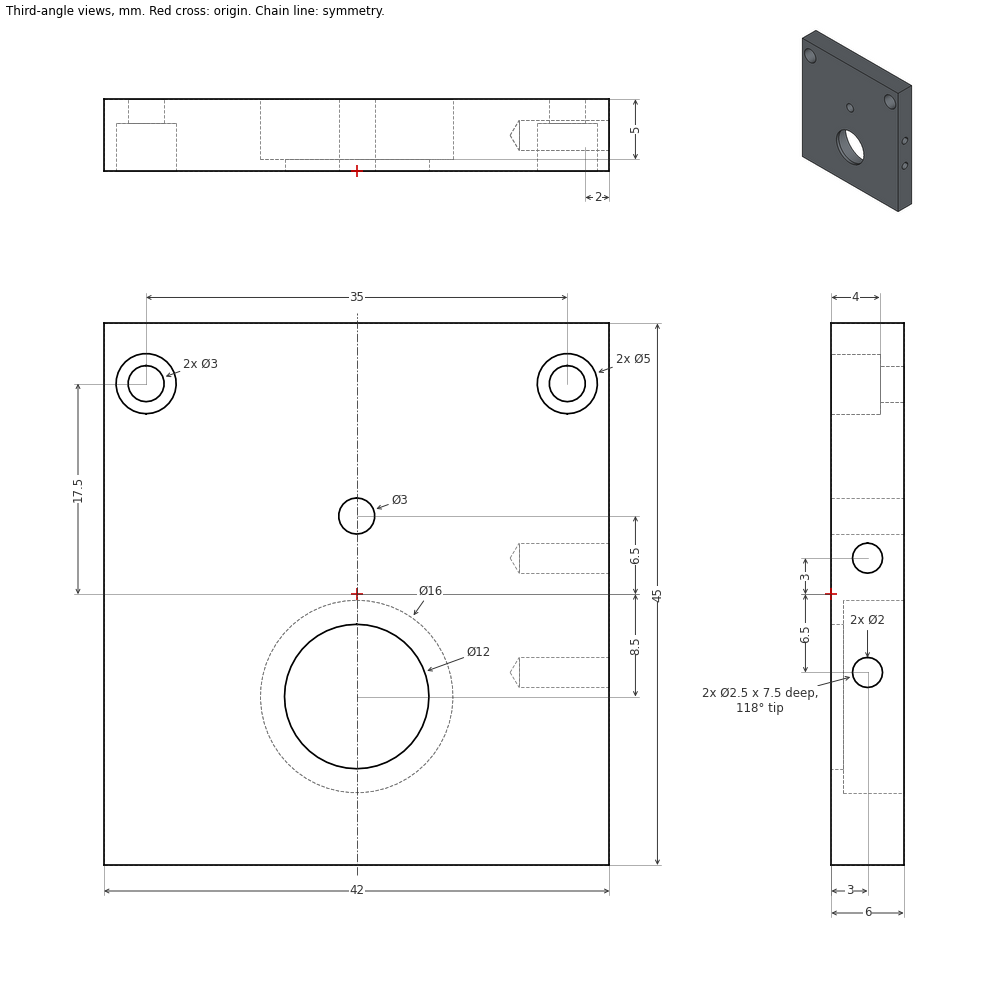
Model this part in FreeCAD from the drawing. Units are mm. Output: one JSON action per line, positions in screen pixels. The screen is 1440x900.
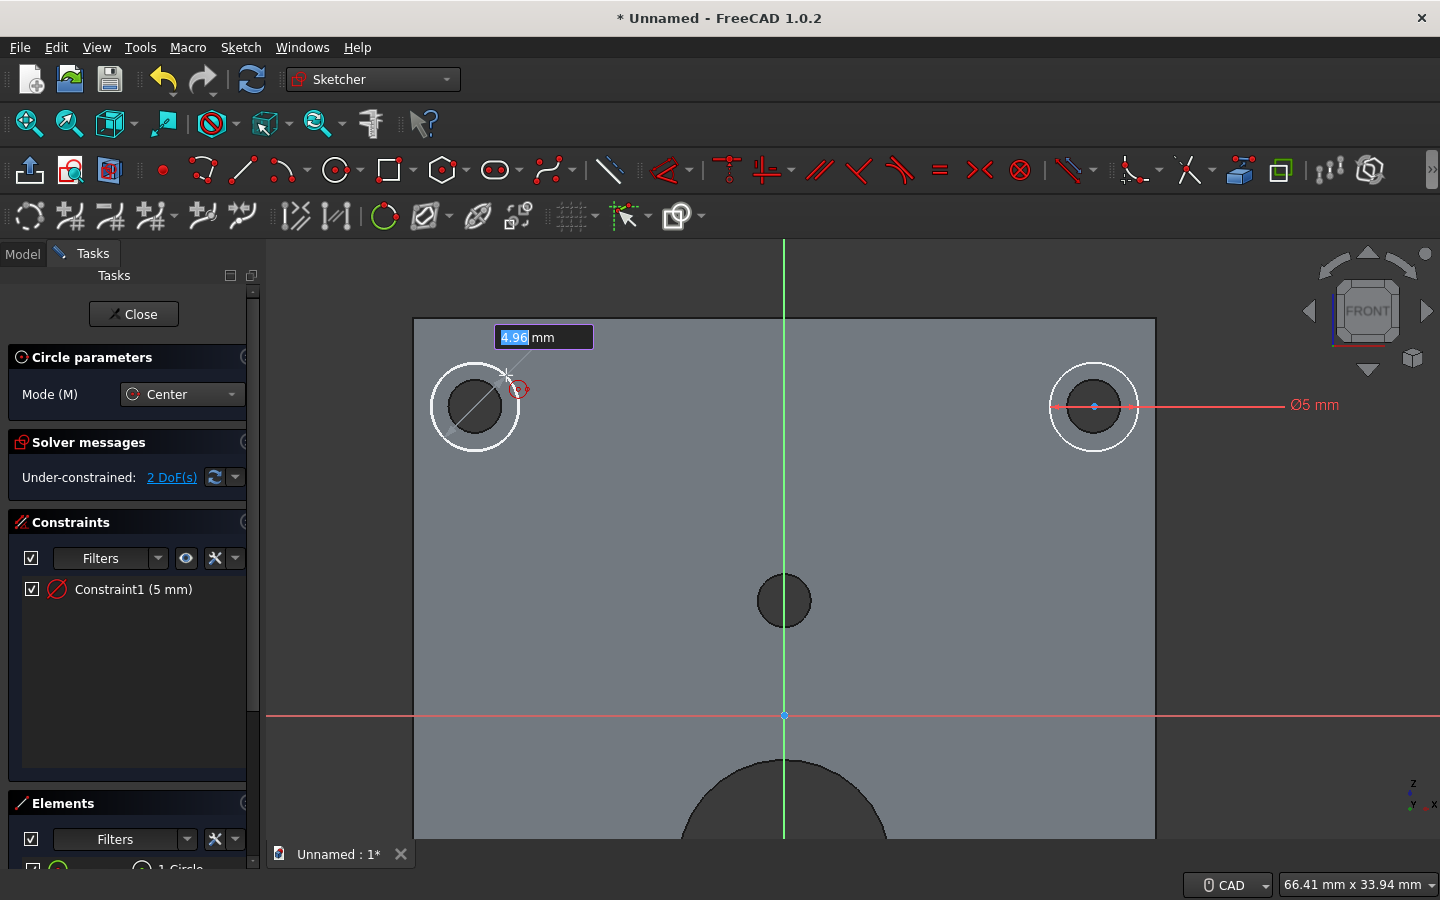
{"action": "type", "text": "5"}
{"action": "key", "text": "Return"}
{"action": "key", "text": "Escape"}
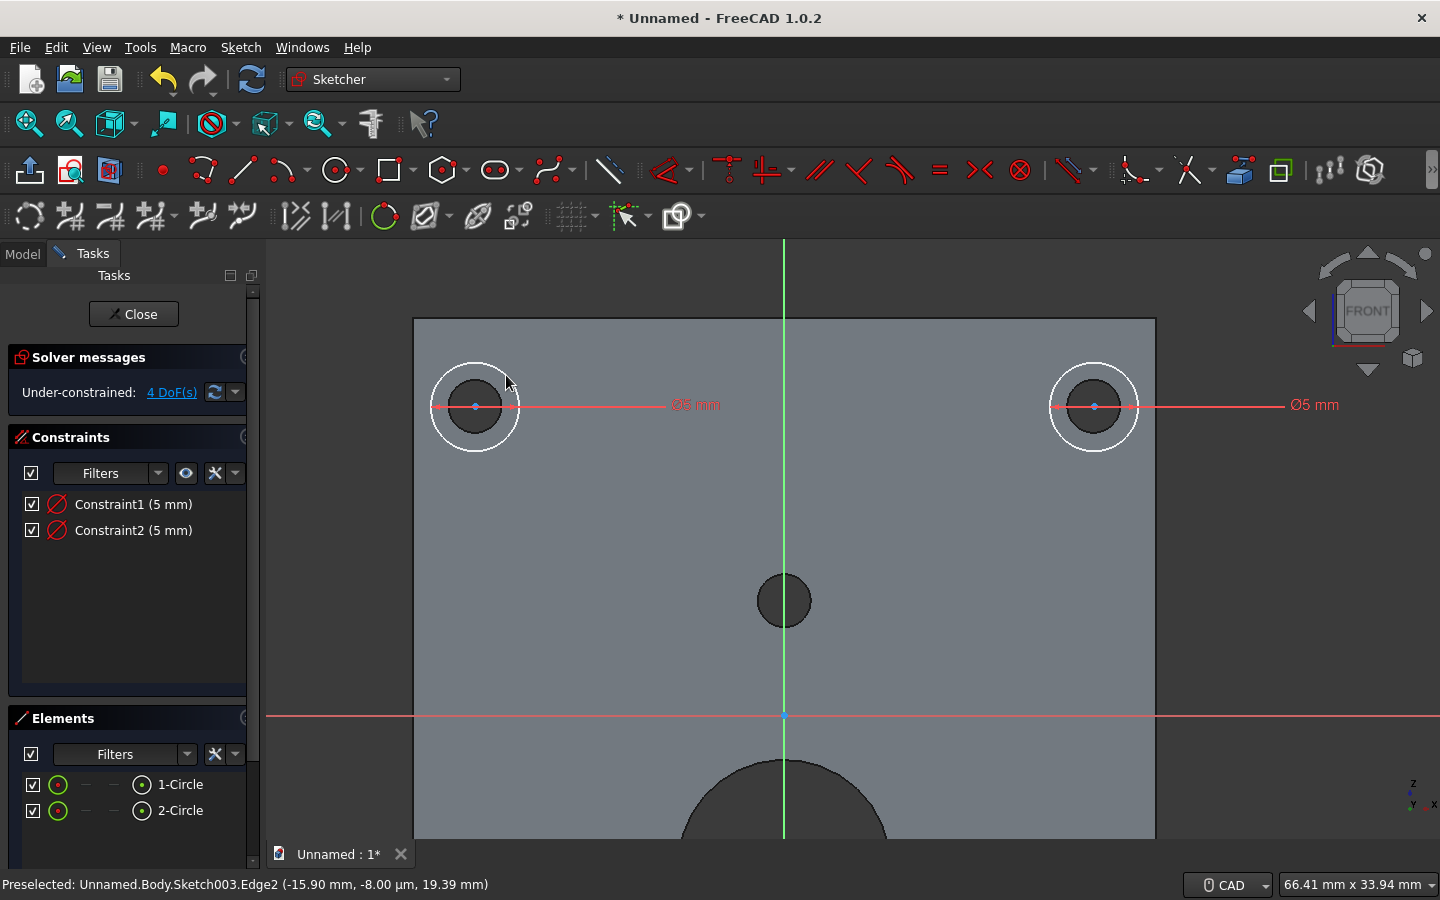
{"action": "left_click", "coordinate": [1094, 407]}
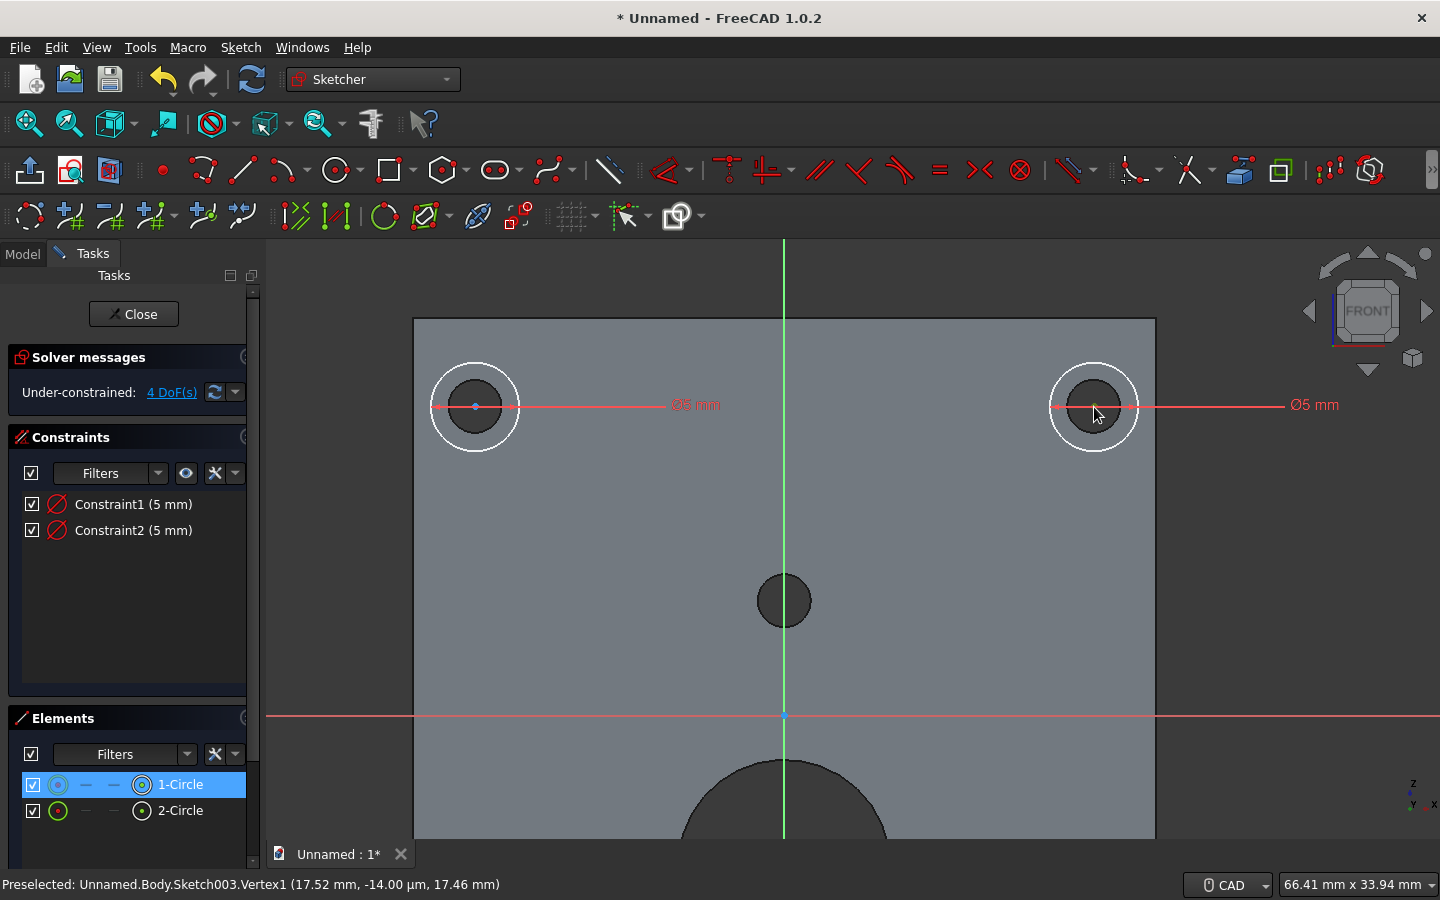
{"action": "left_click", "coordinate": [475, 407]}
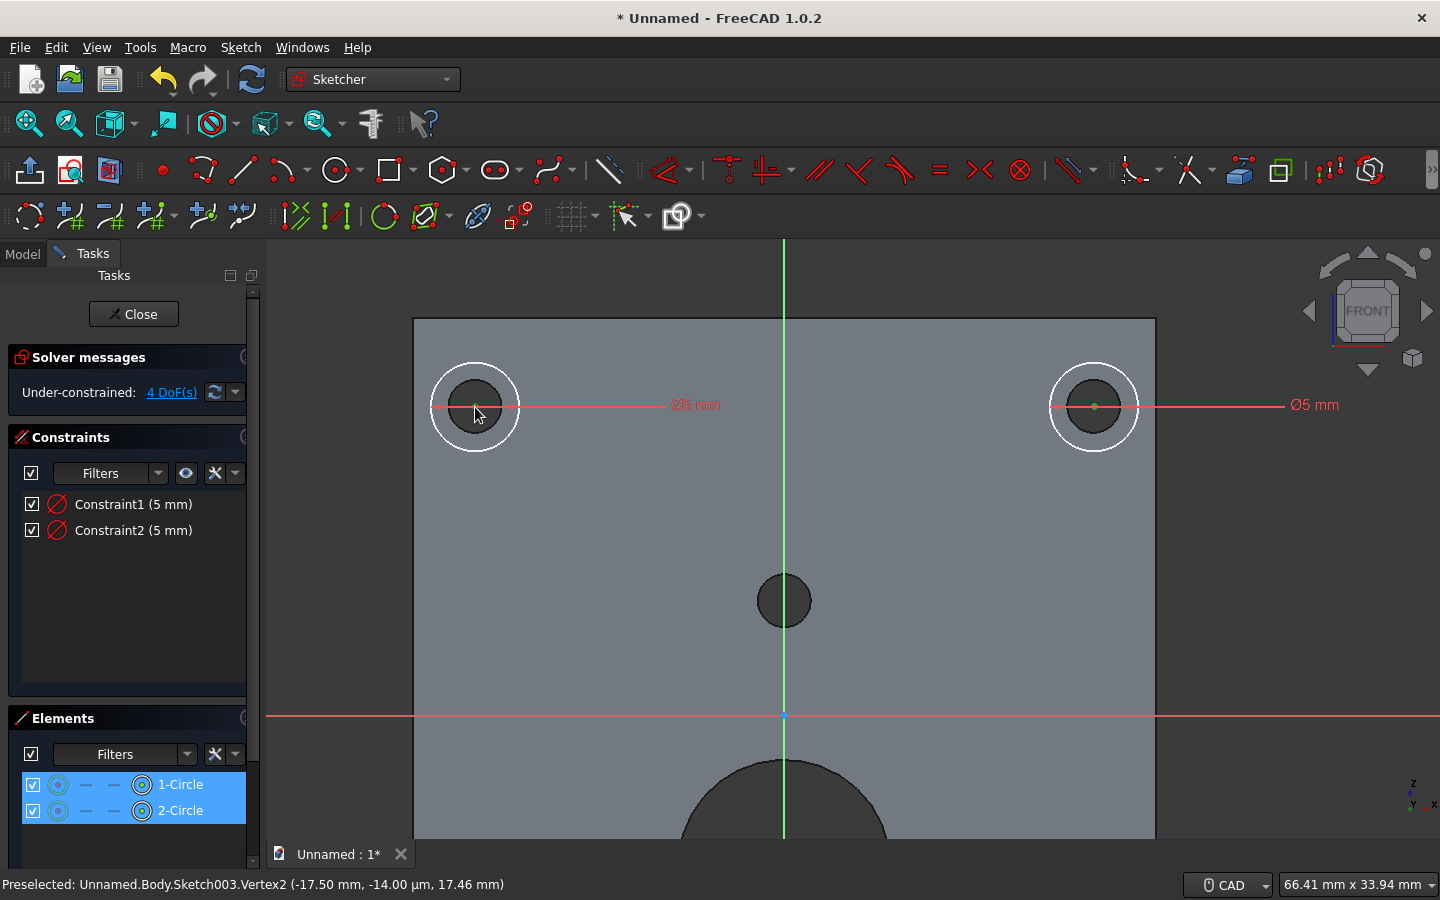
{"action": "left_click", "coordinate": [784, 772]}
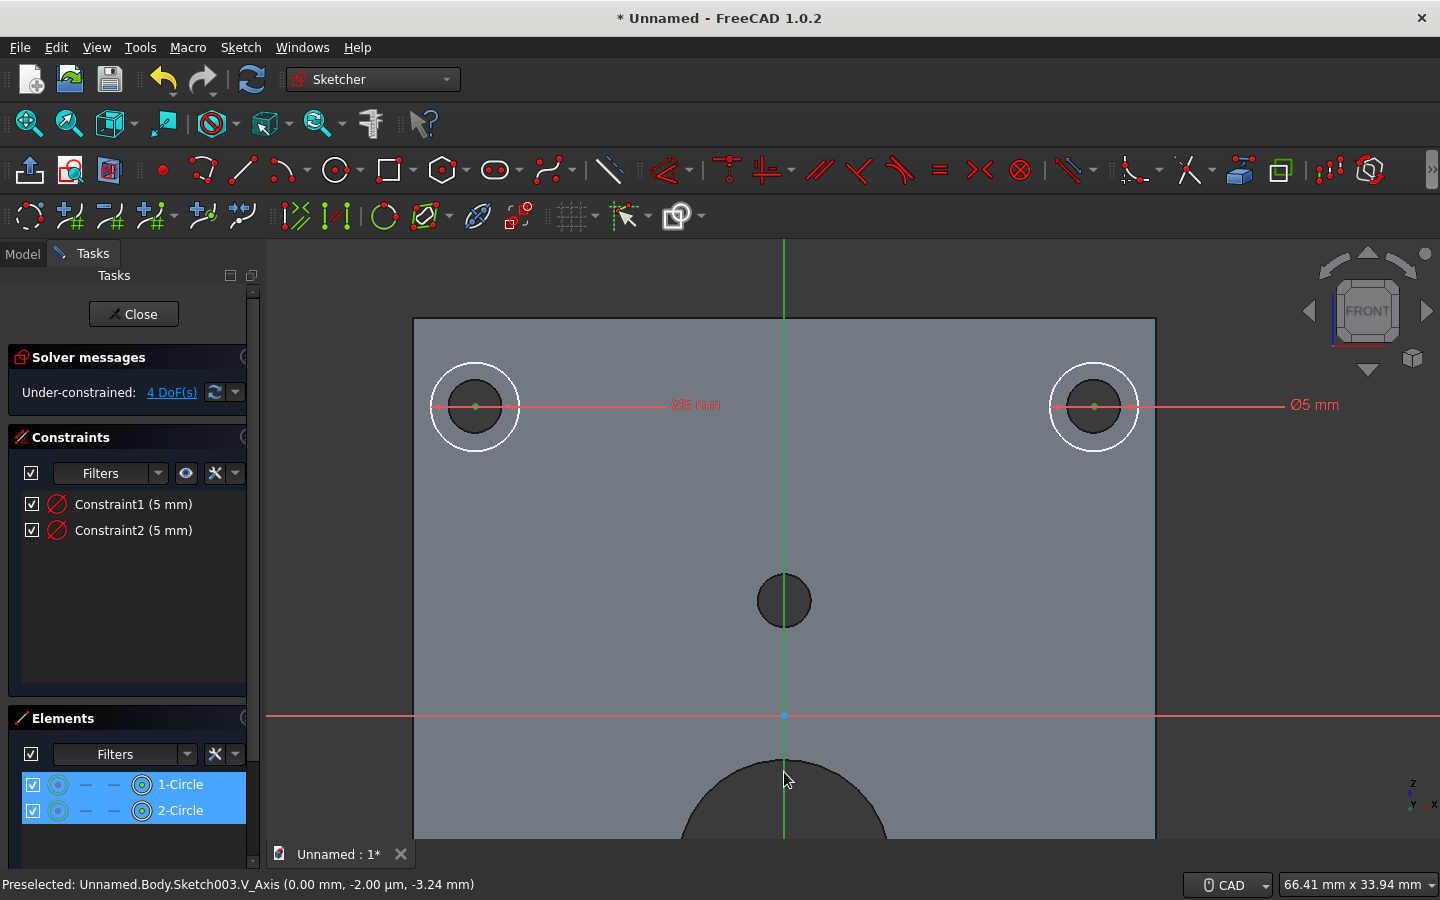
{"action": "key", "text": "s"}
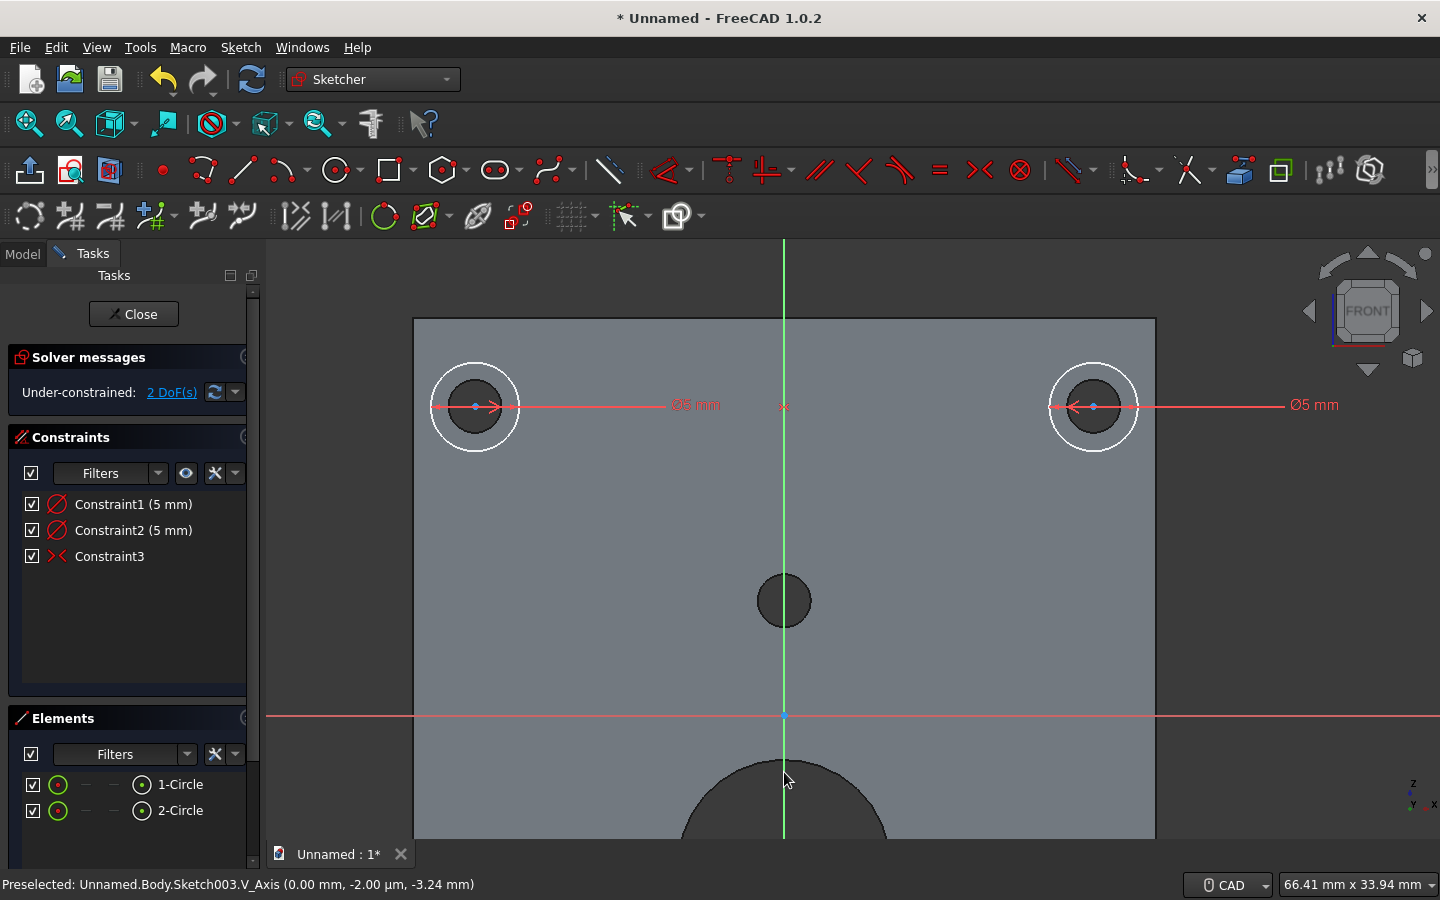
{"action": "key", "text": "d"}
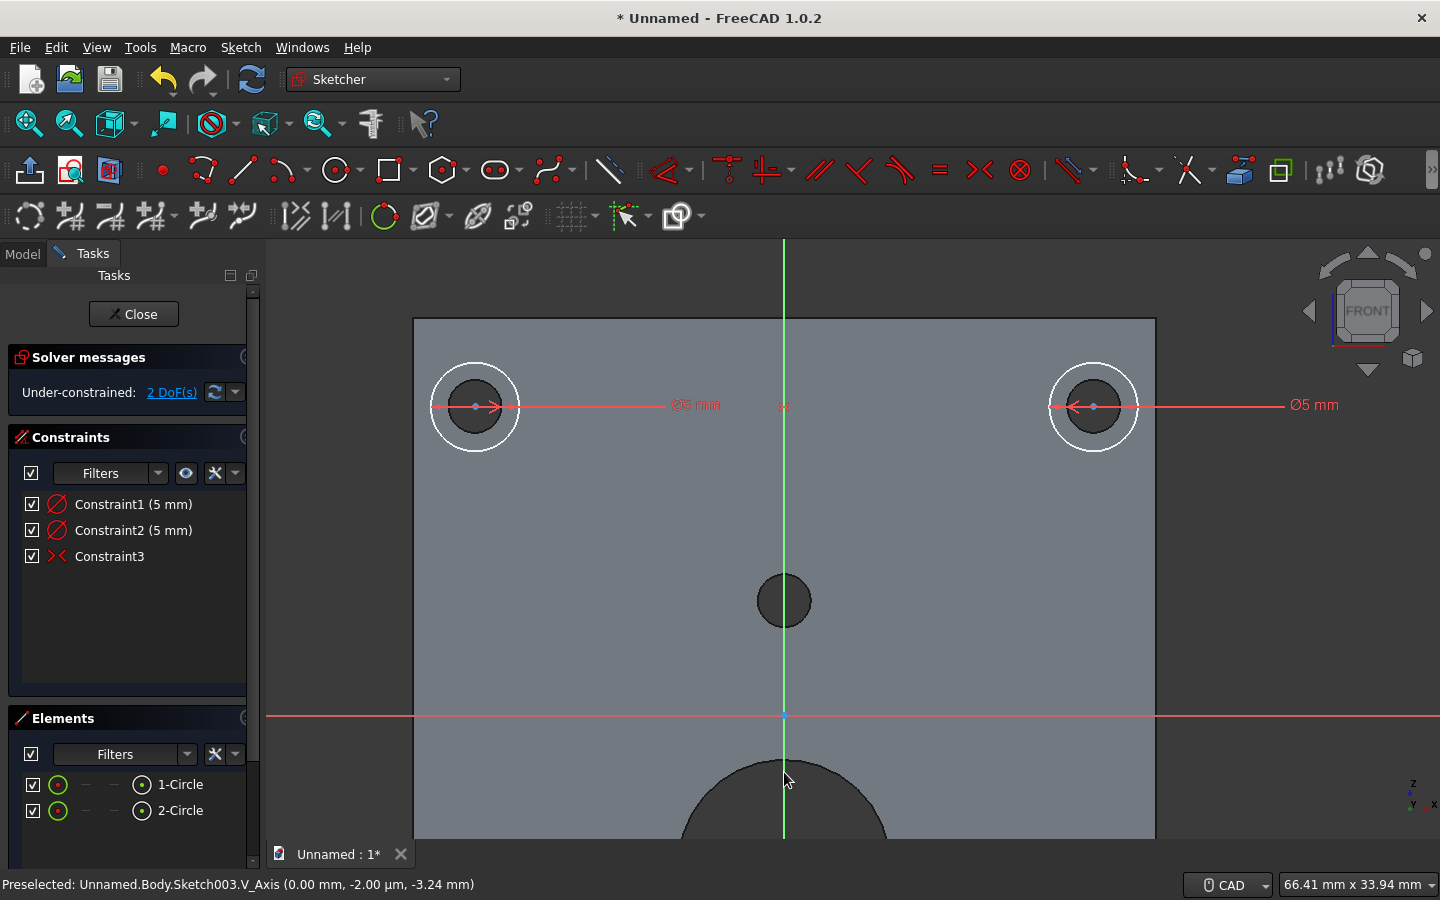
{"action": "left_click", "coordinate": [1094, 407]}